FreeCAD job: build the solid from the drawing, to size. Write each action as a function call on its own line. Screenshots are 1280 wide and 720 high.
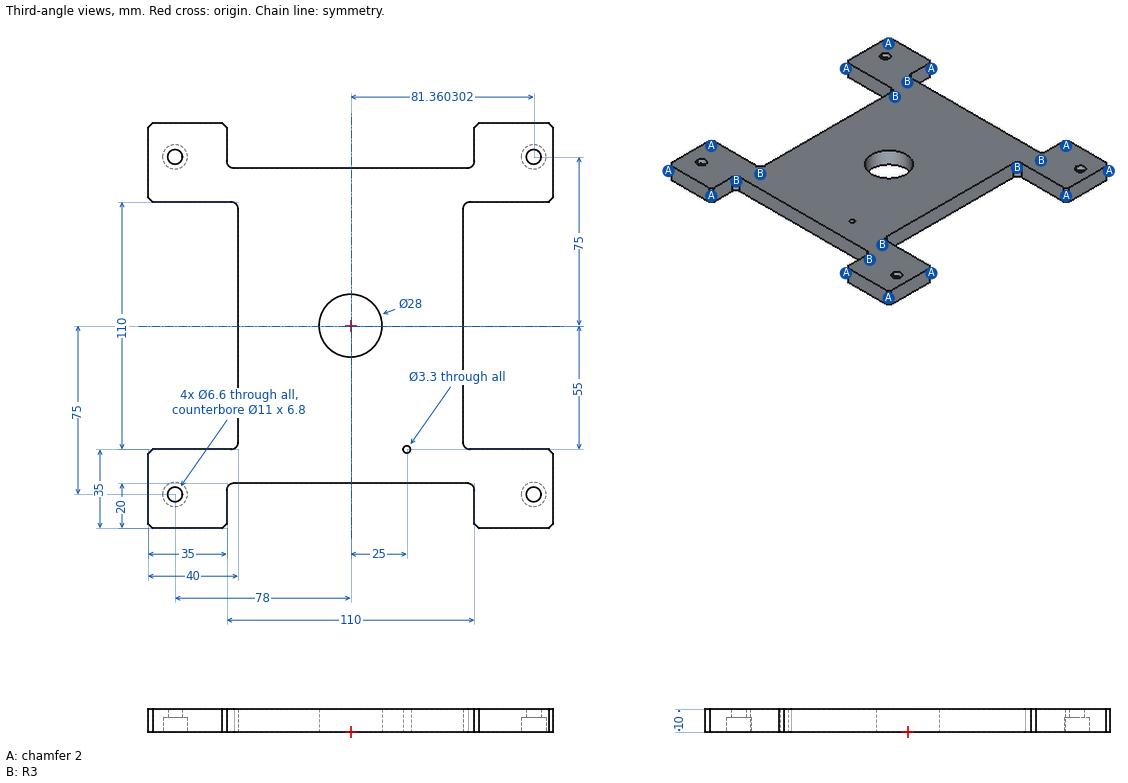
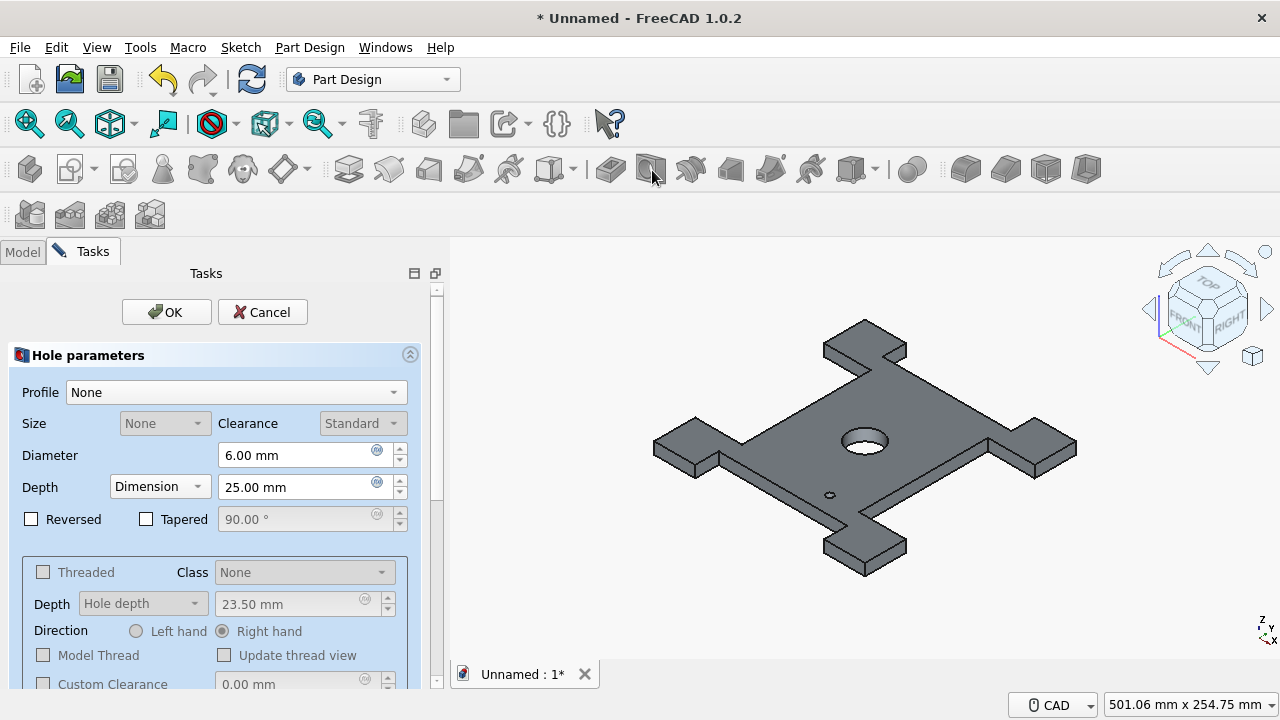
triple_click(305, 455)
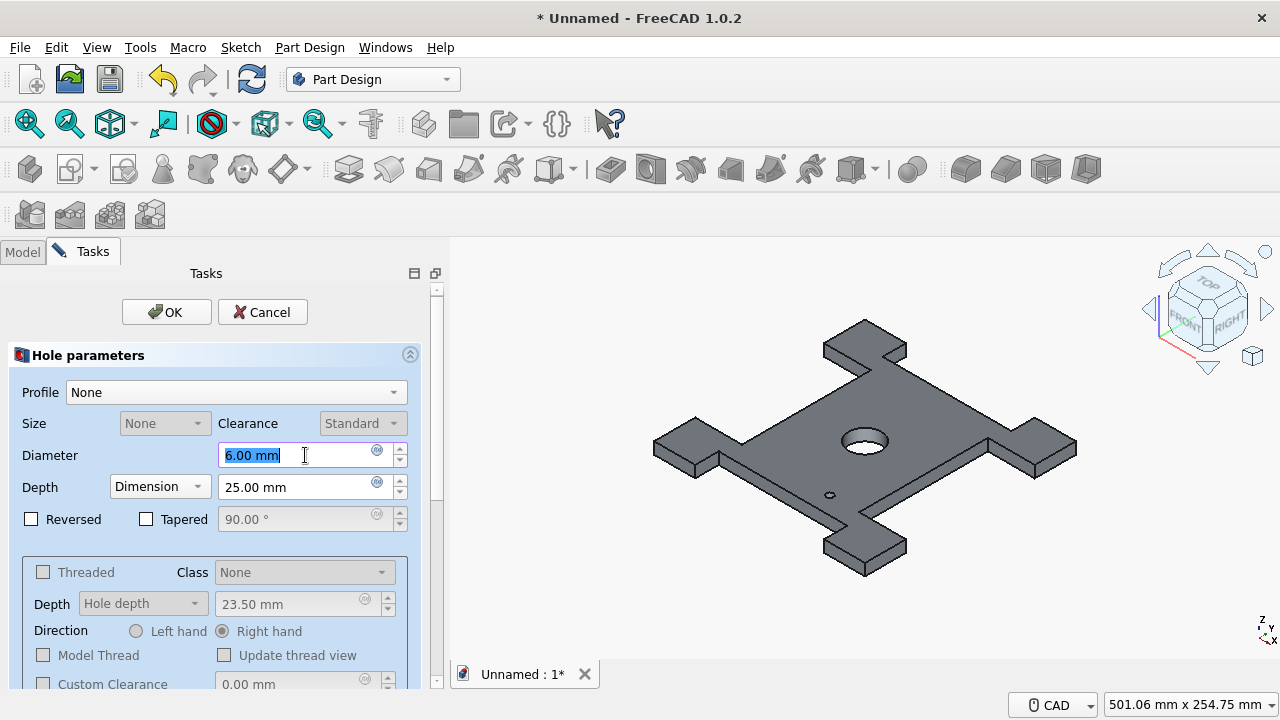
text(3.3)
key(Tab)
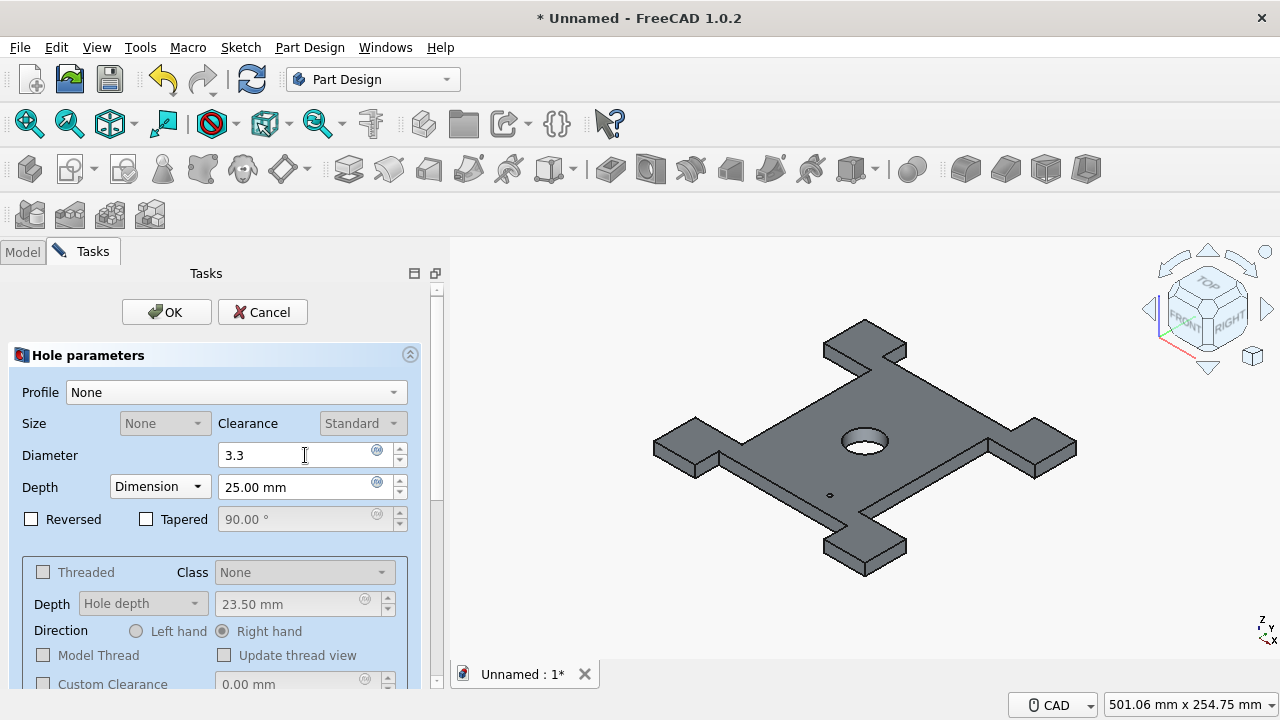
click(161, 486)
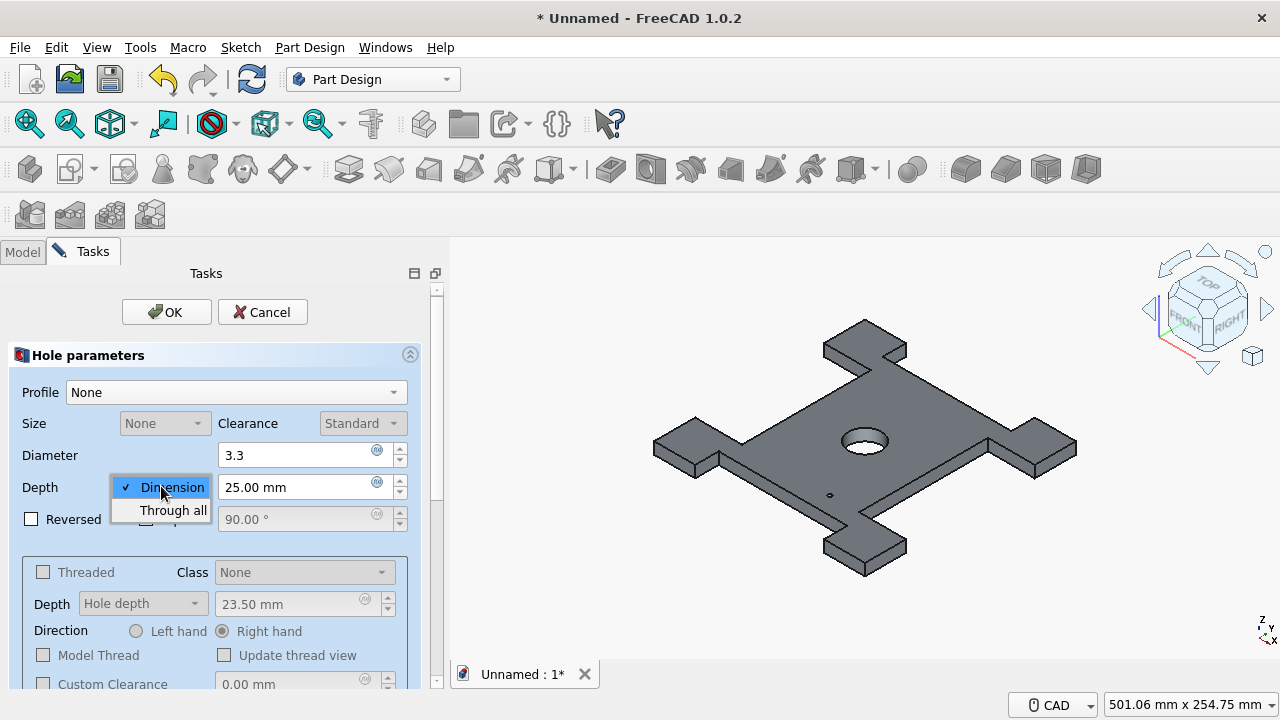
click(160, 510)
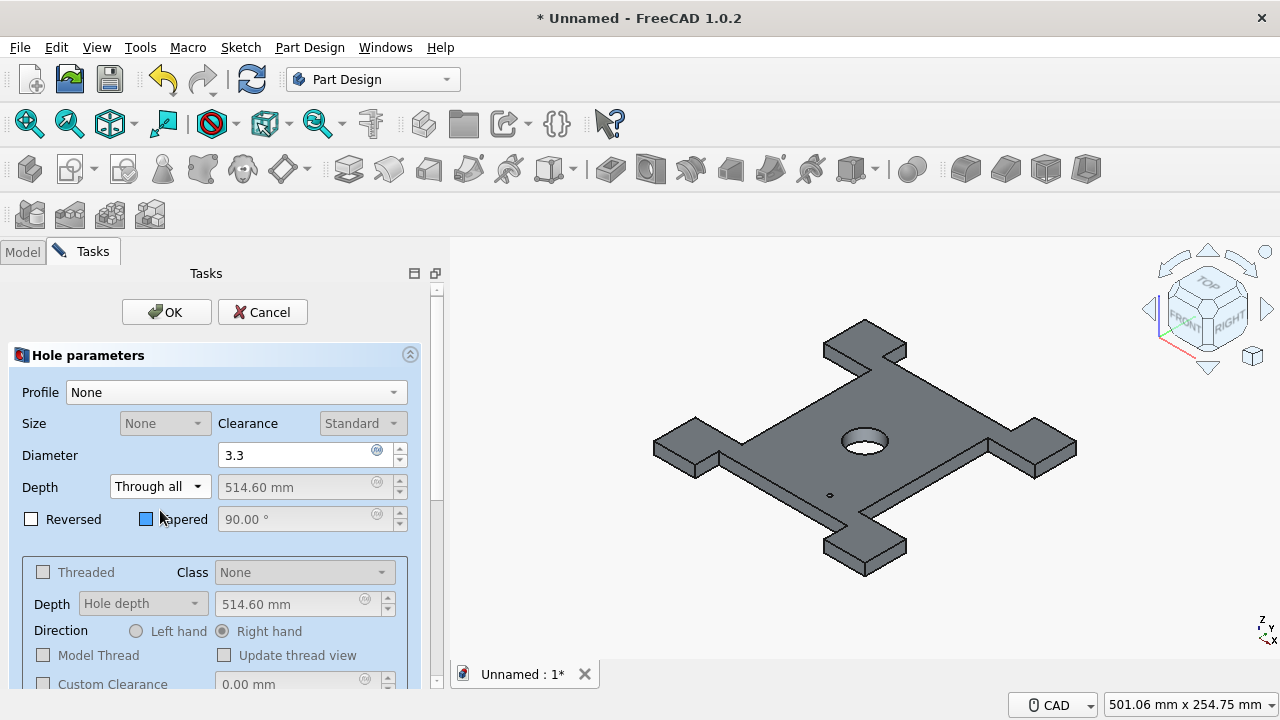
click(167, 312)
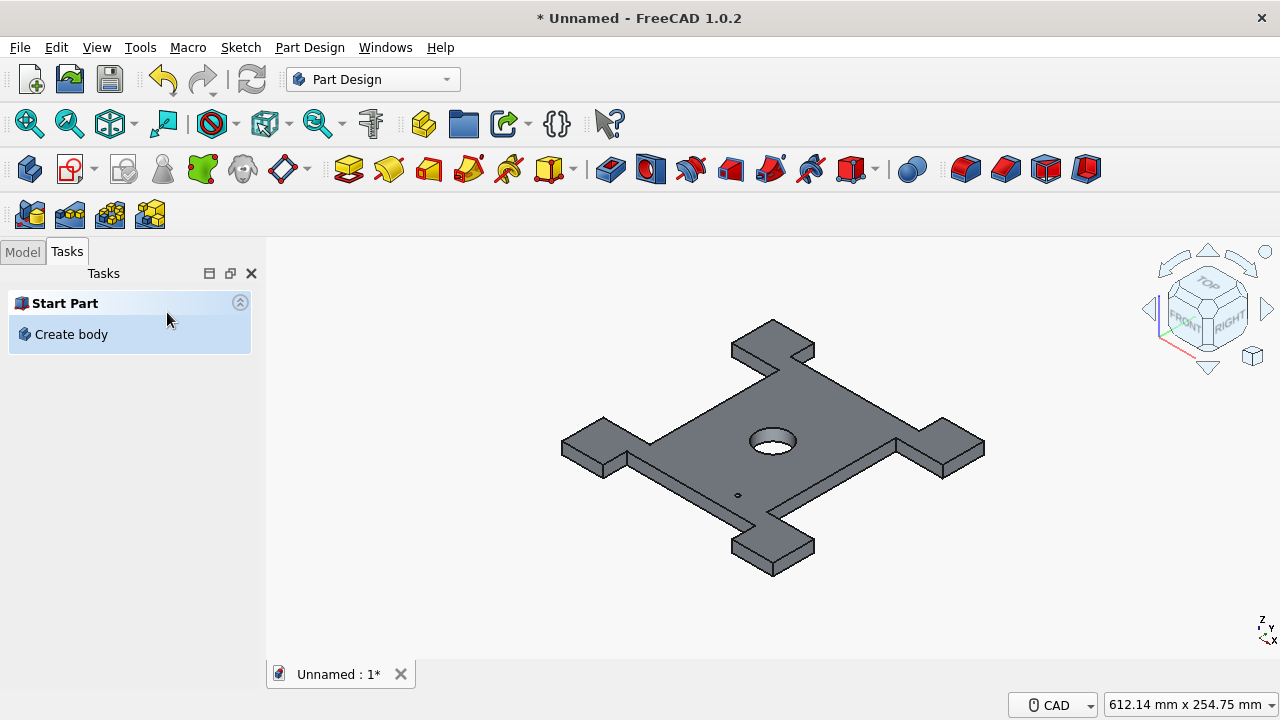
key(5)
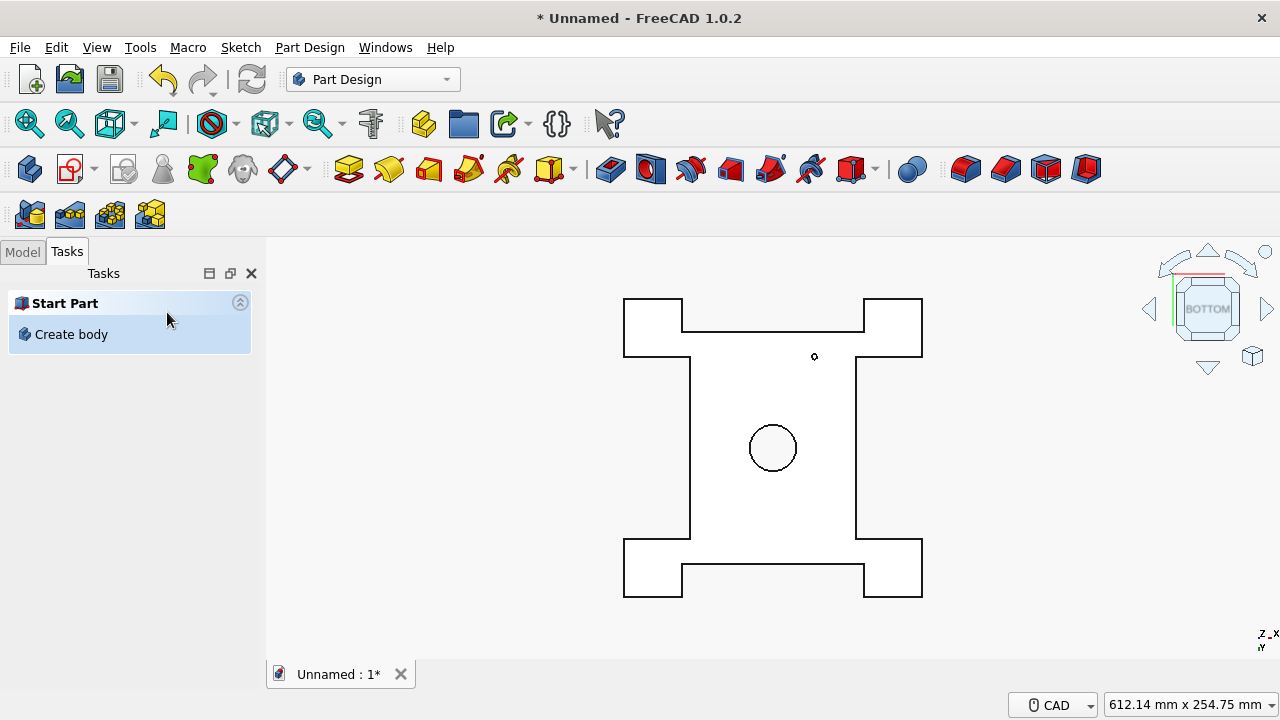
click(816, 490)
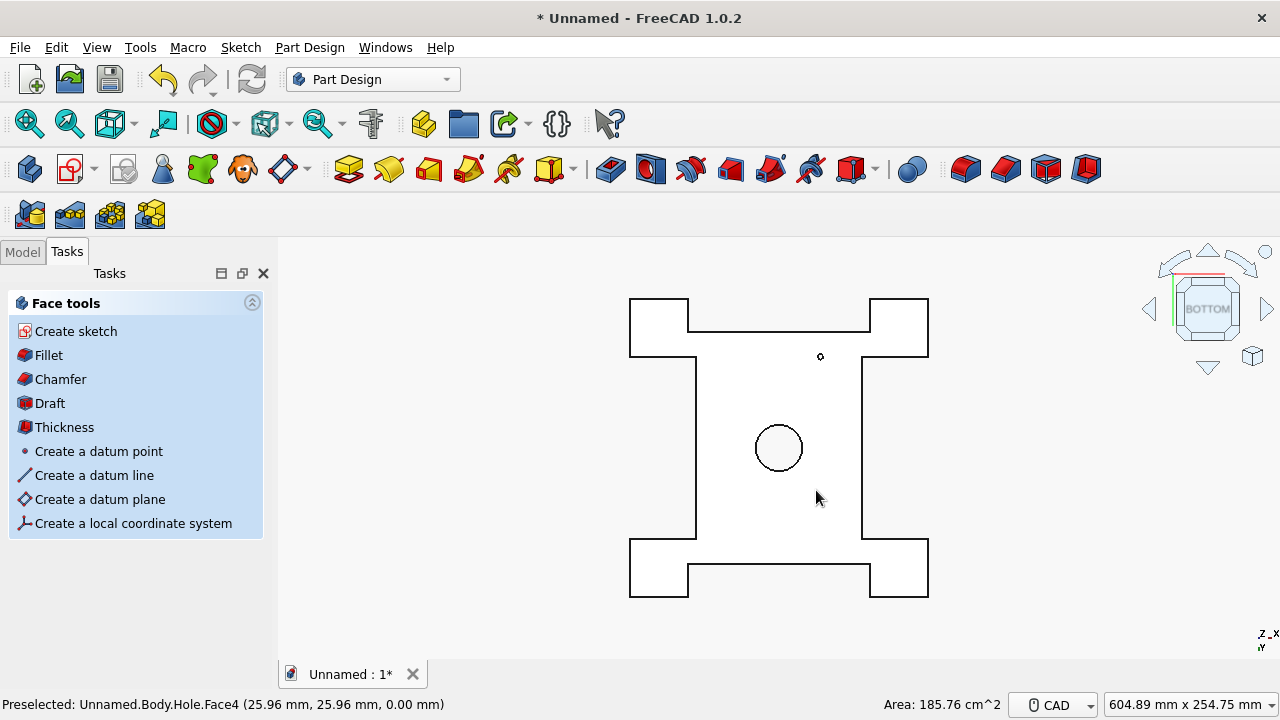
click(70, 170)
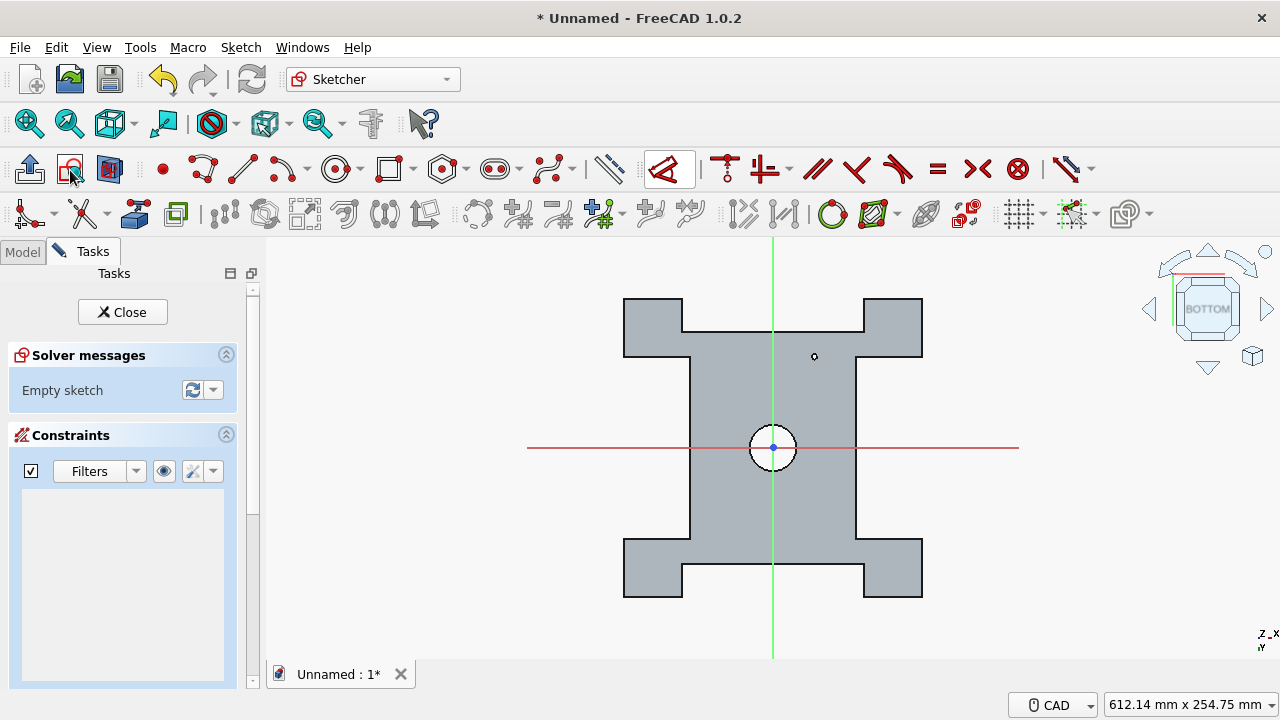
key(g)
key(c)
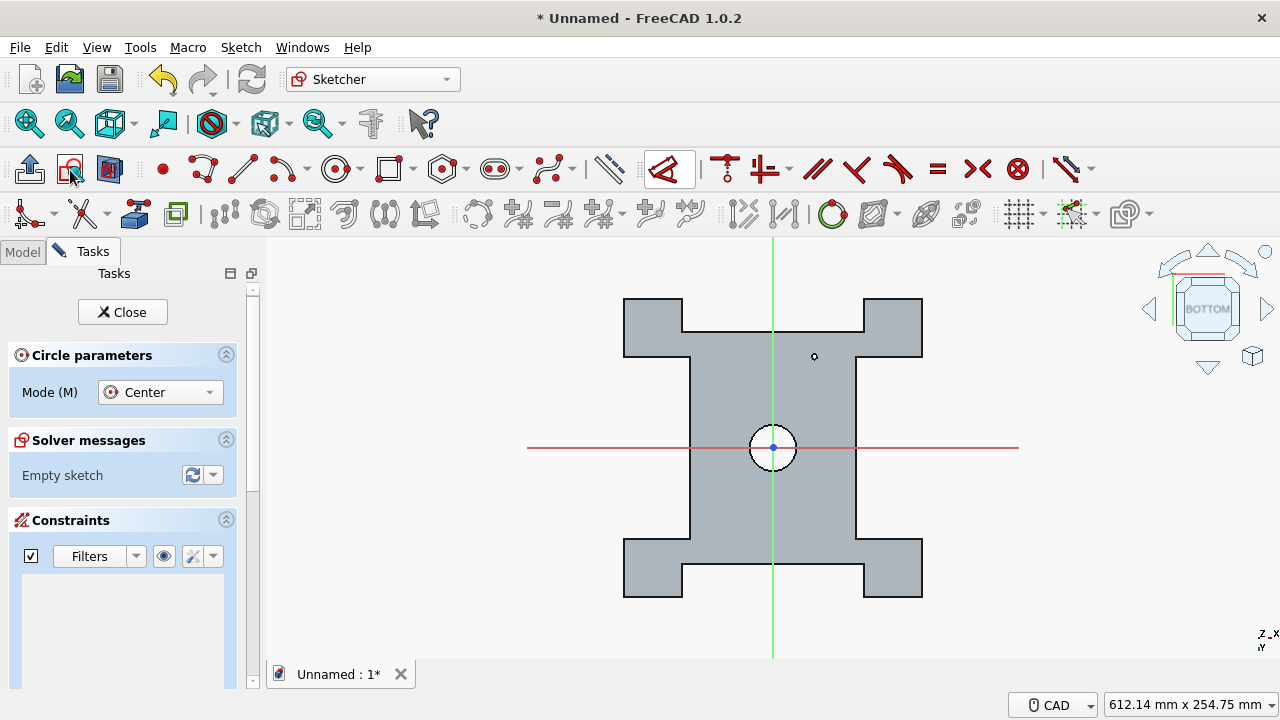
scroll(644, 324, up, 8)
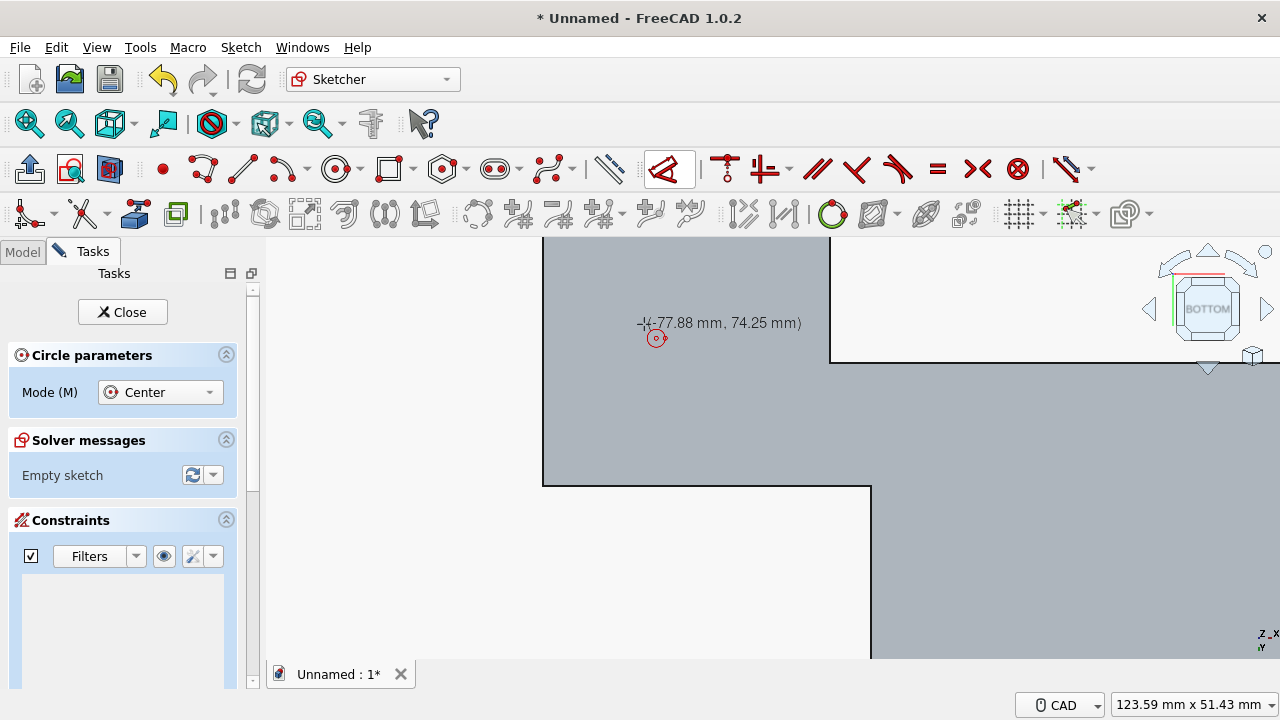
scroll(555, 324, down, 8)